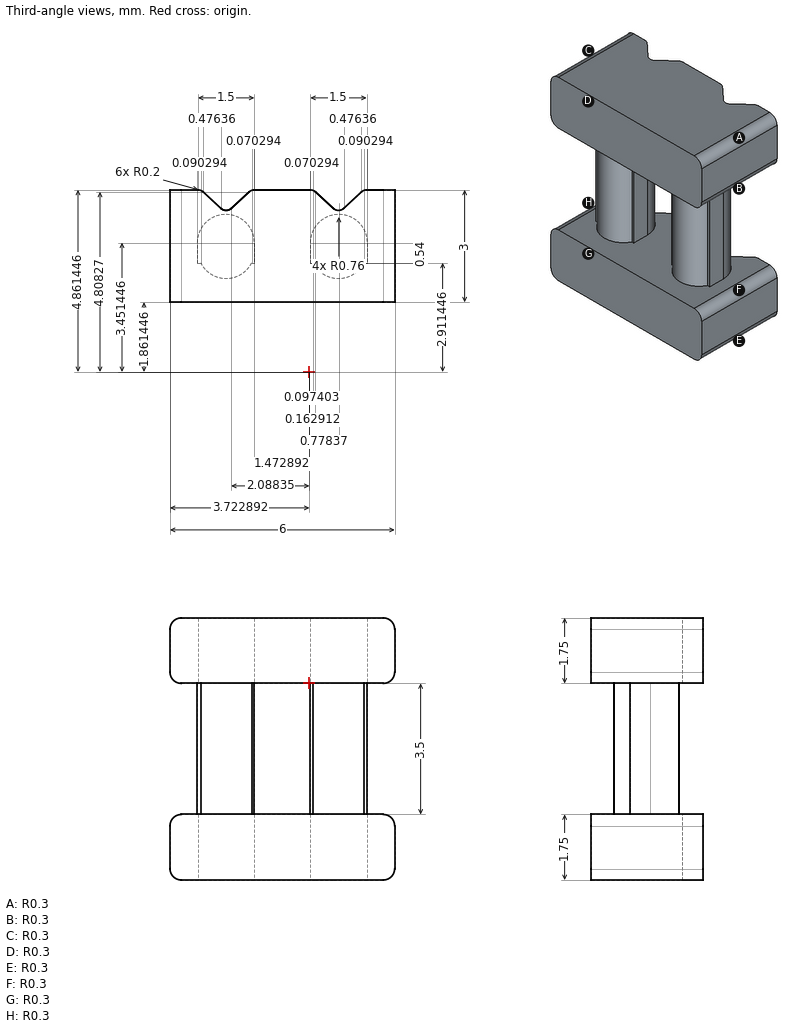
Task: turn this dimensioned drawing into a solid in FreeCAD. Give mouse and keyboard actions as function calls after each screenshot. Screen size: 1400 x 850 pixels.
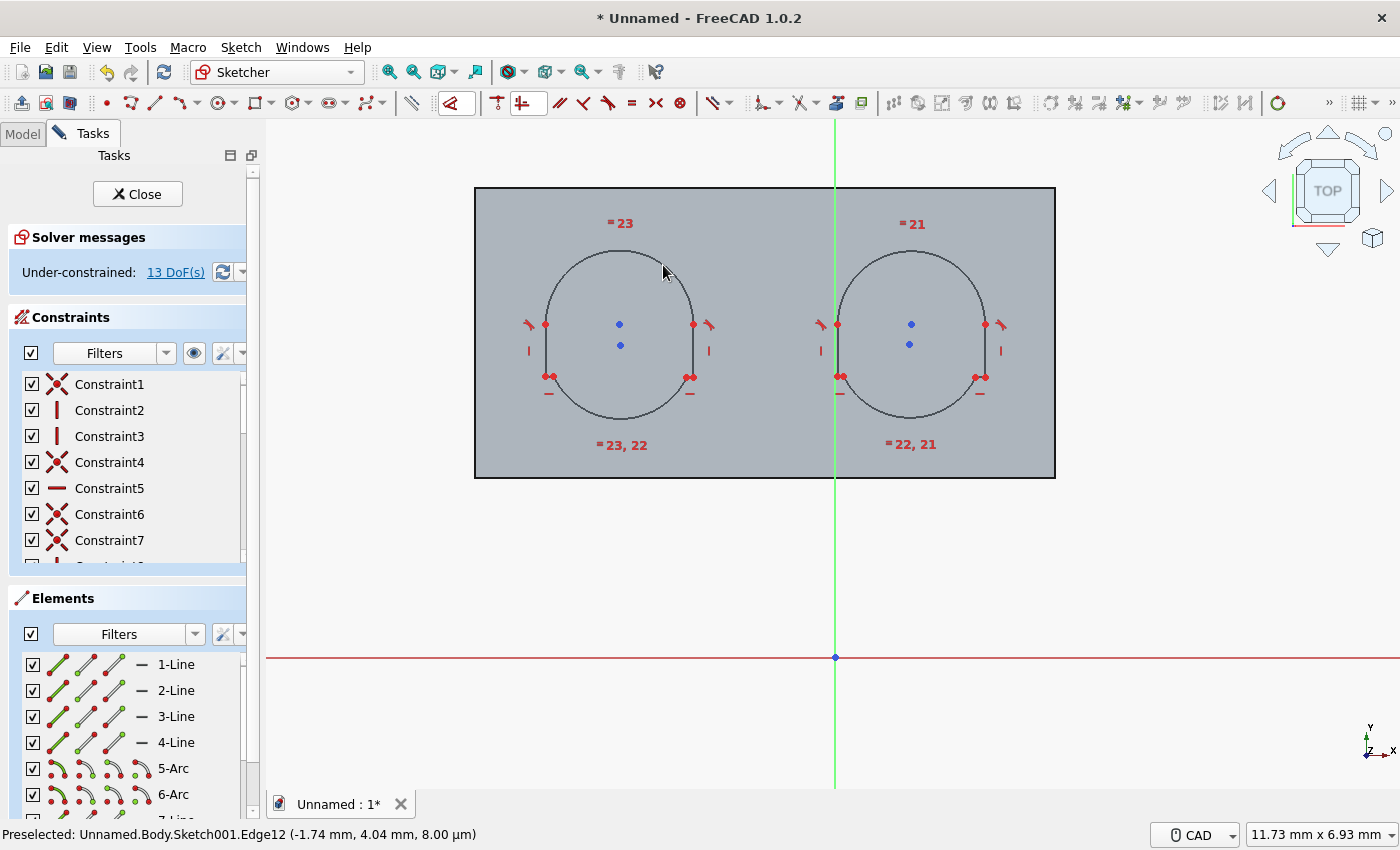
click(955, 265)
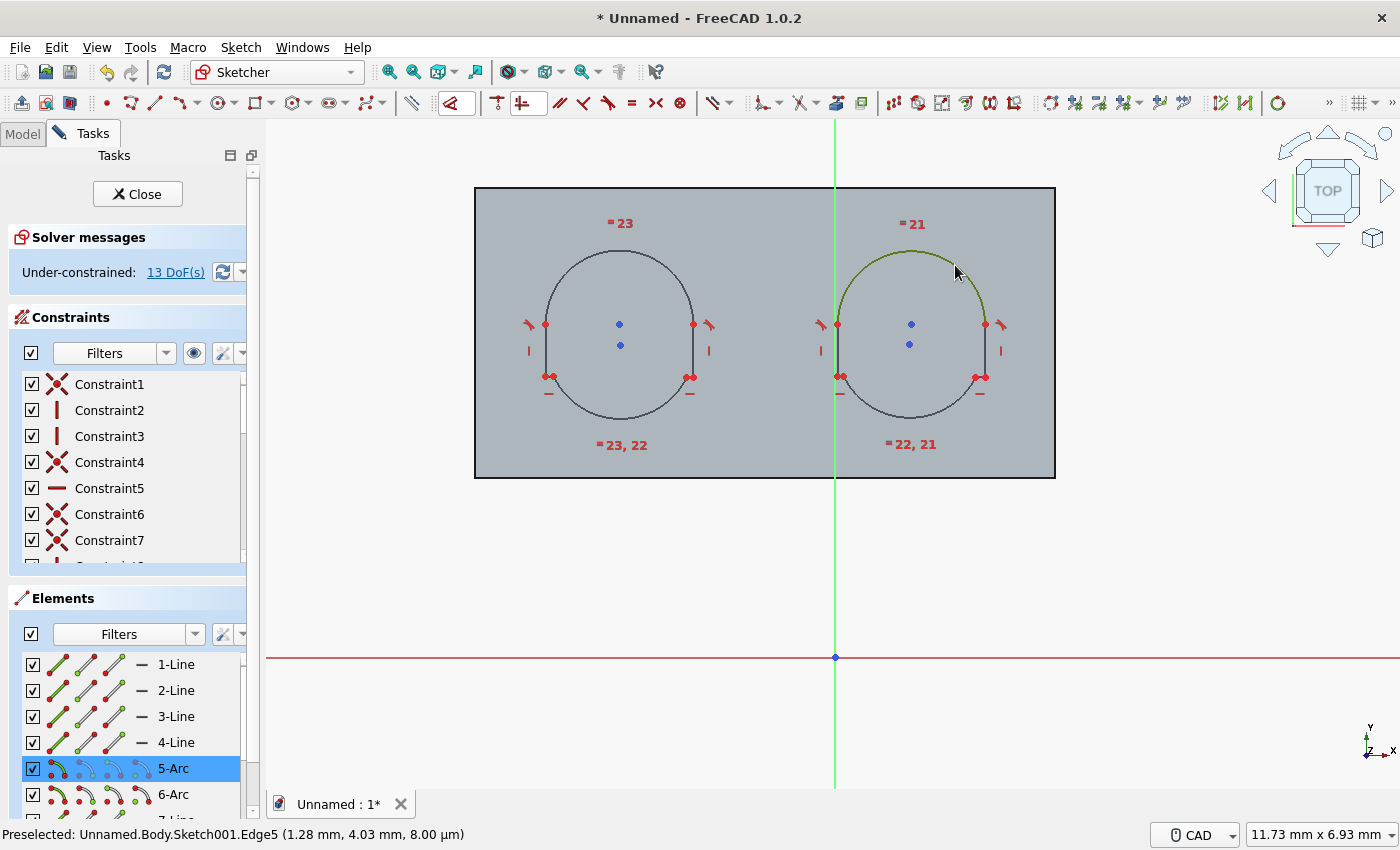
key(k)
key(r)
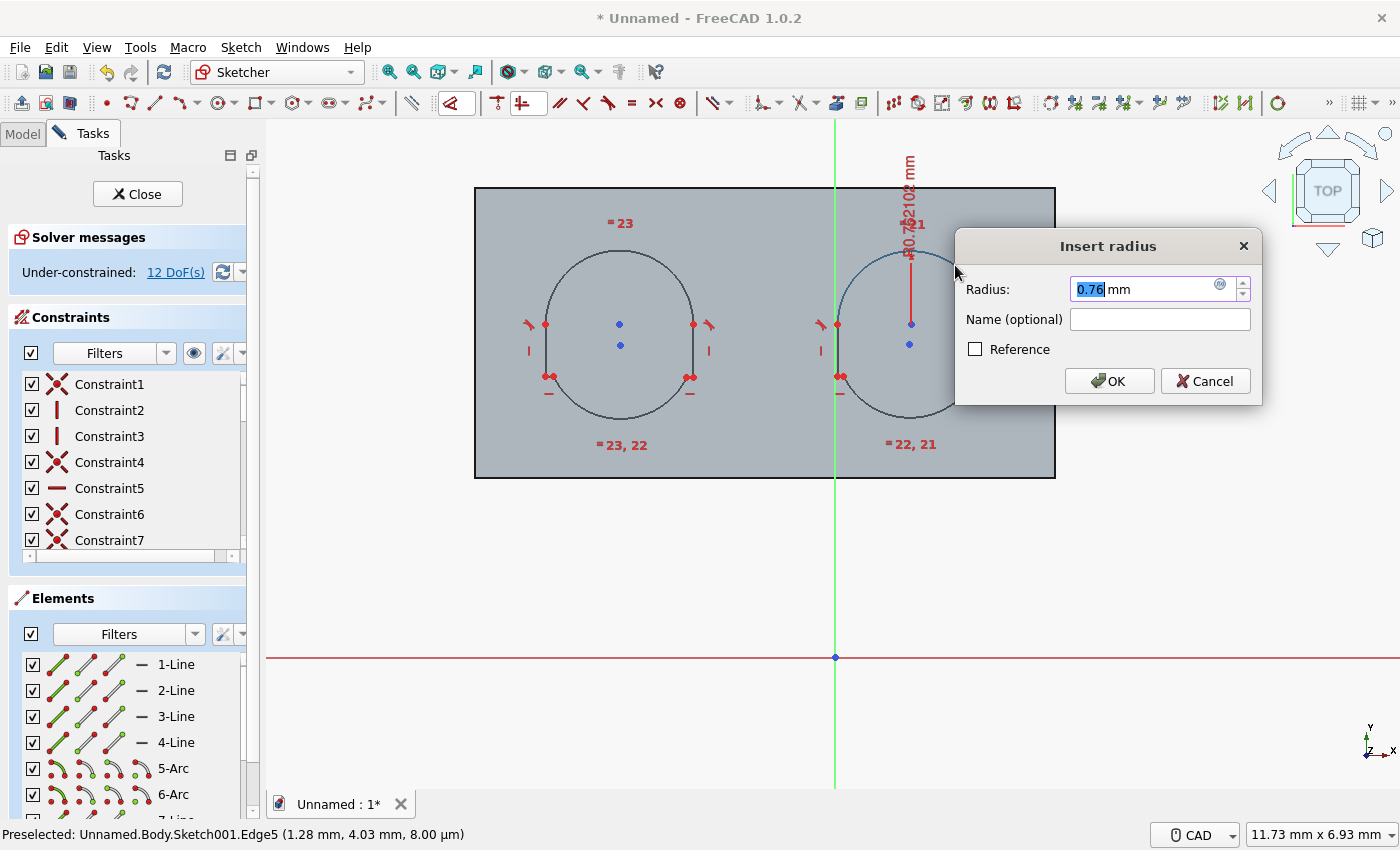
text(0.76)
key(Return)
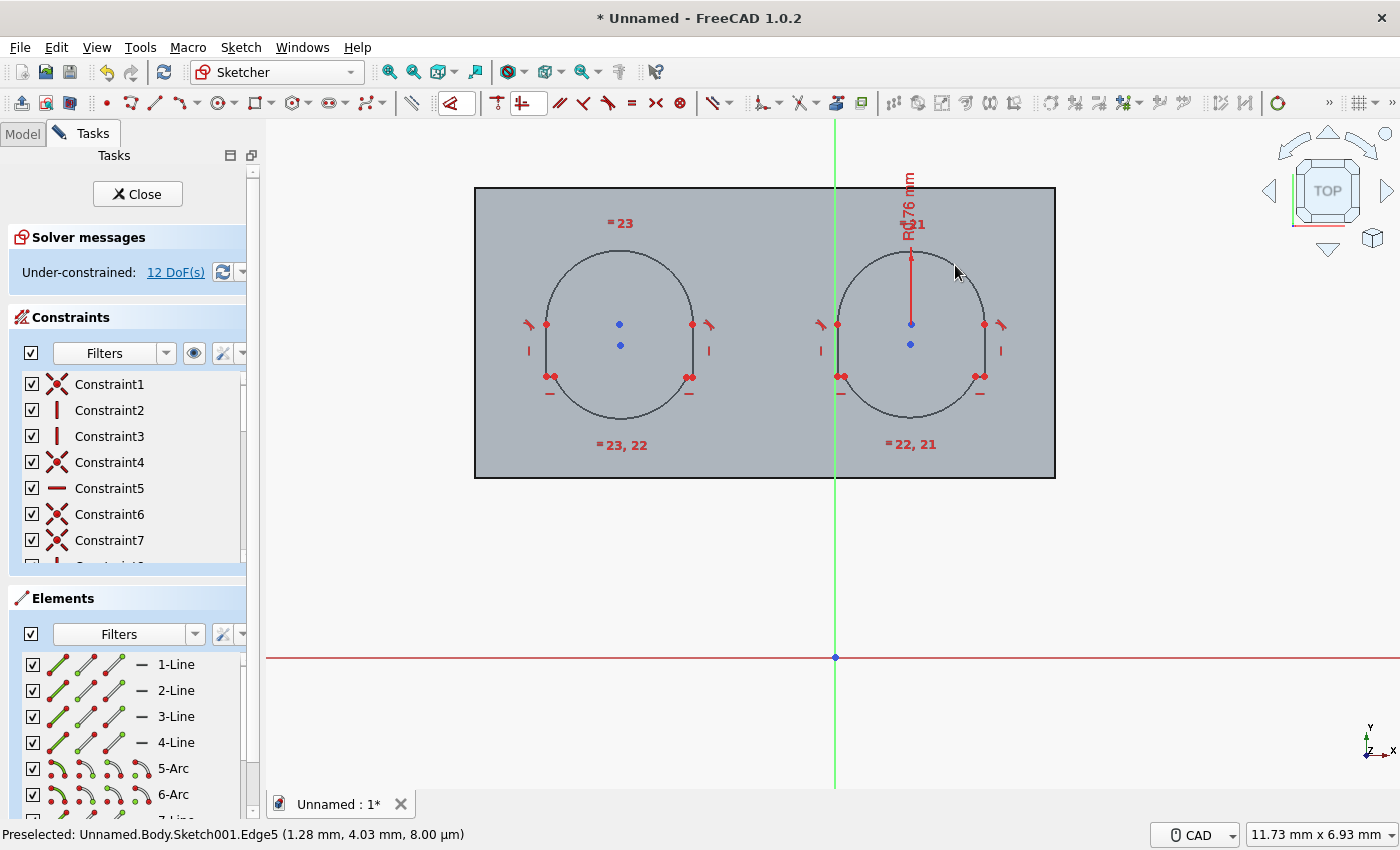
click(838, 361)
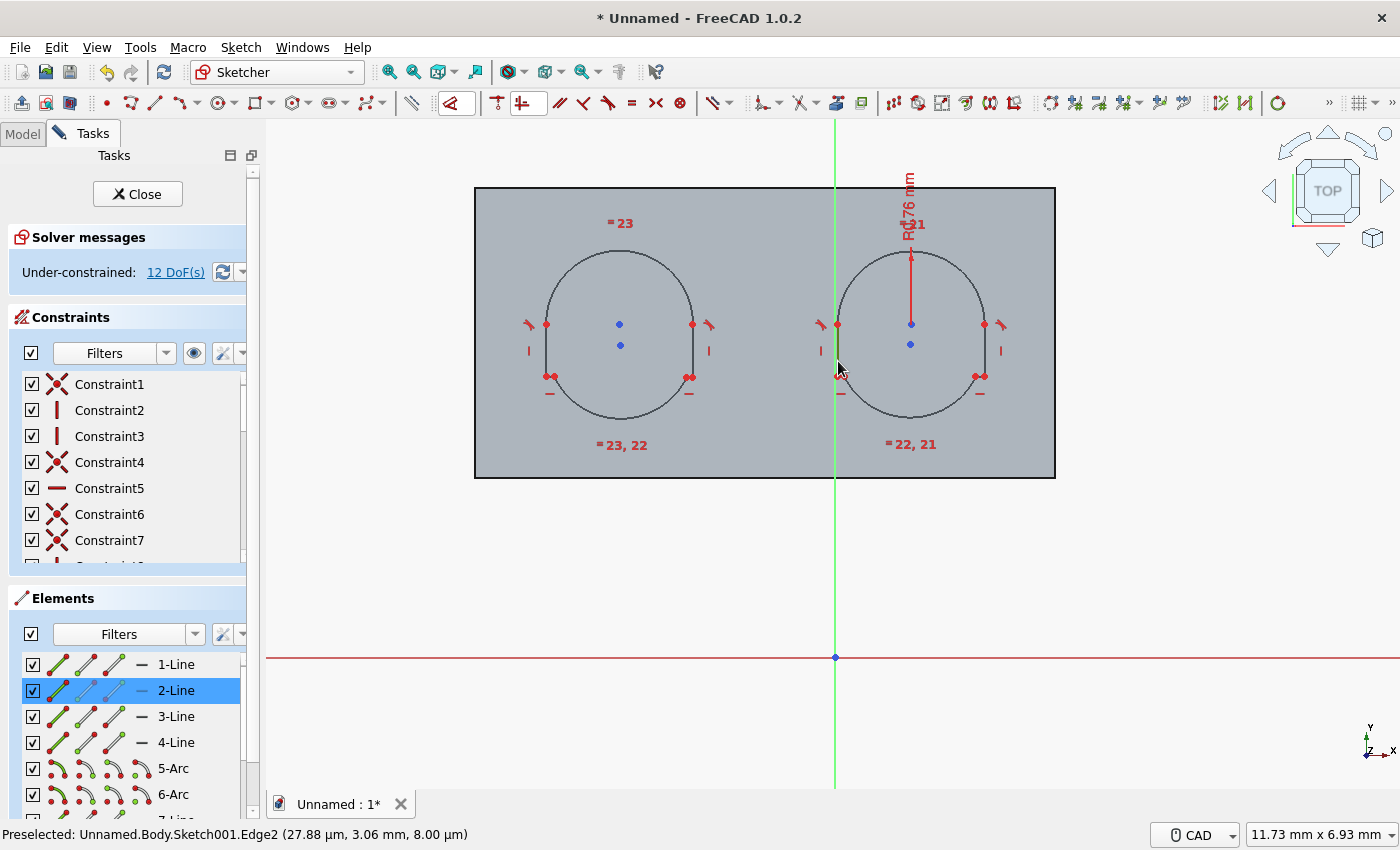
click(470, 104)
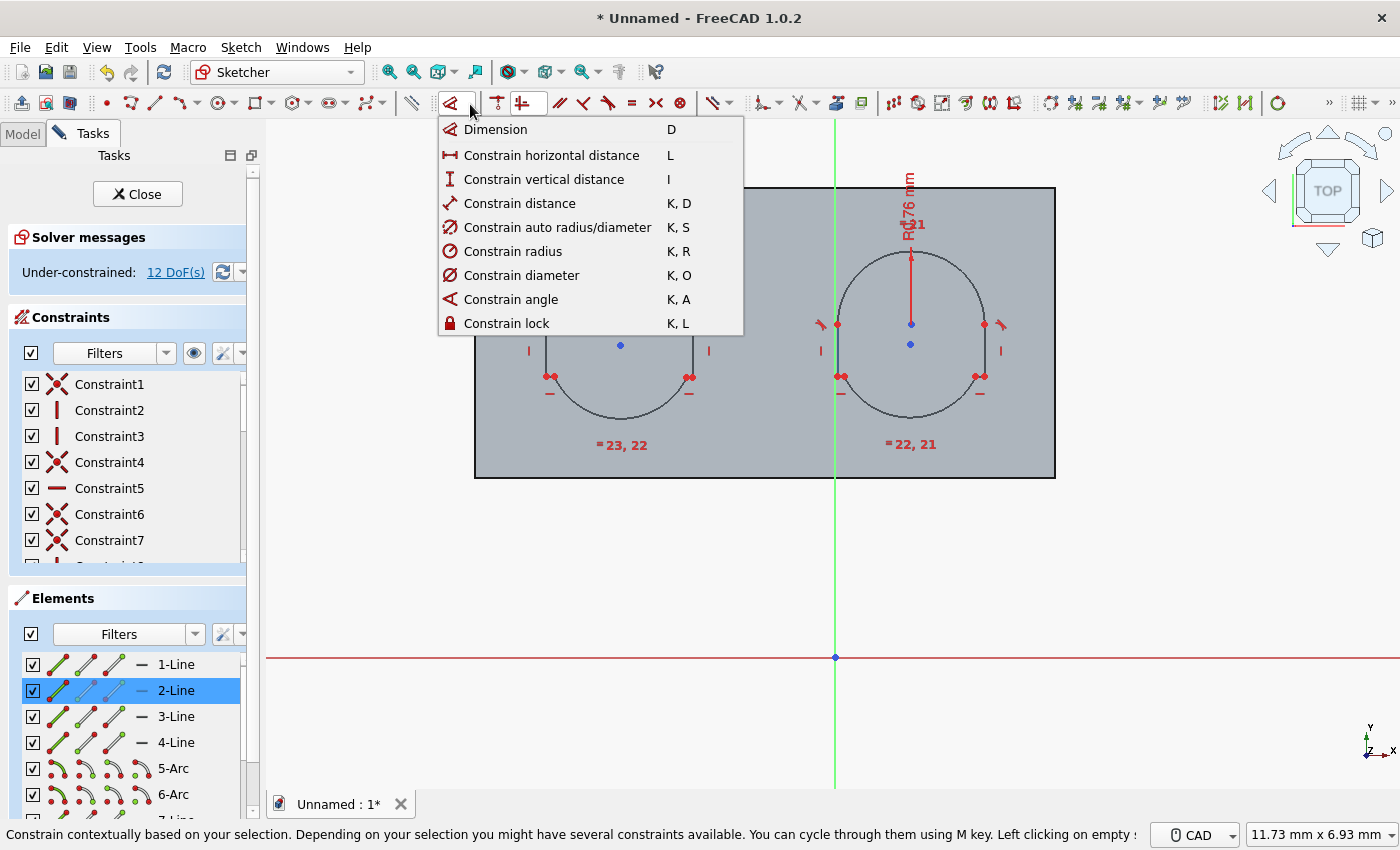
click(591, 179)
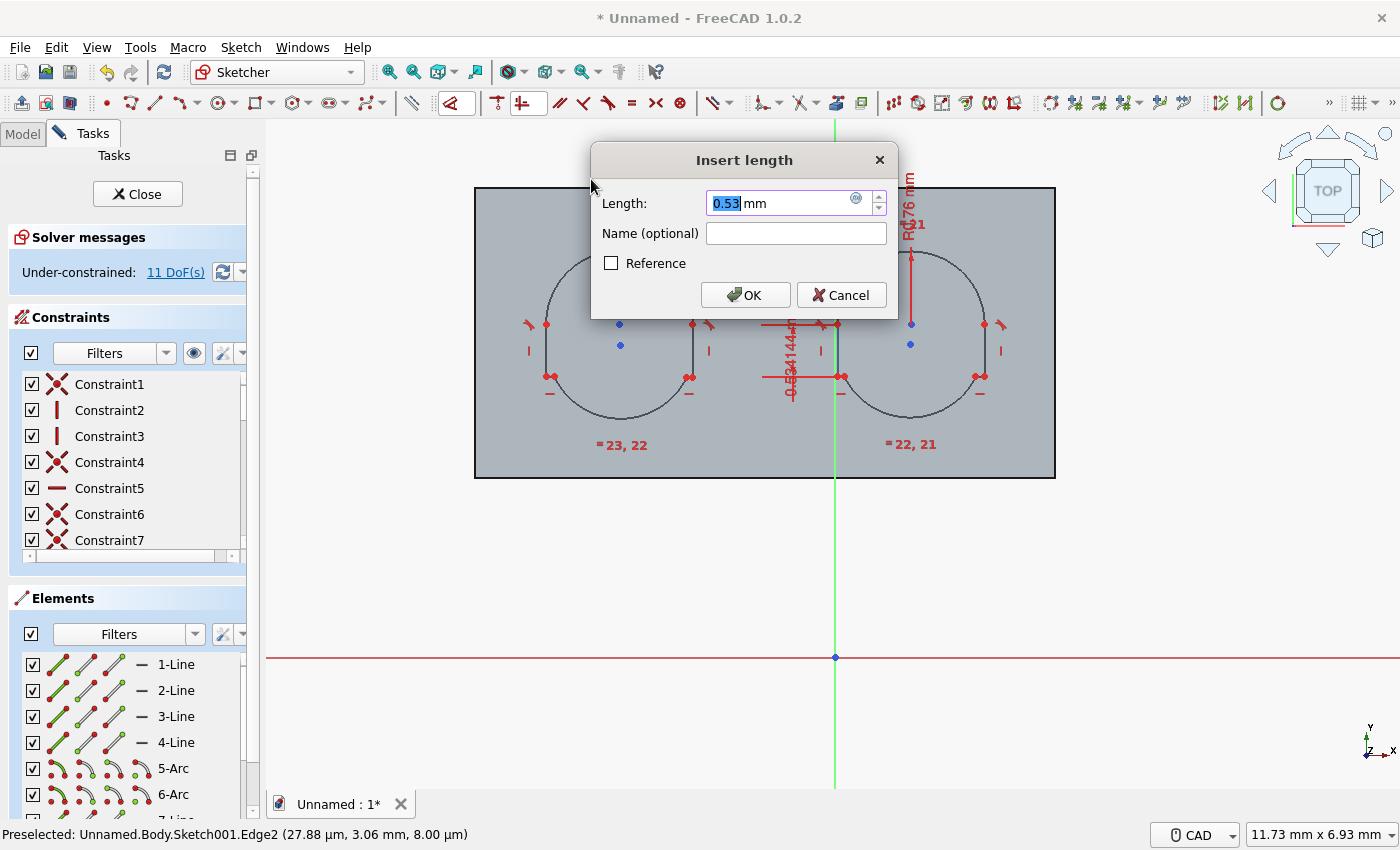
text(0.54)
key(Return)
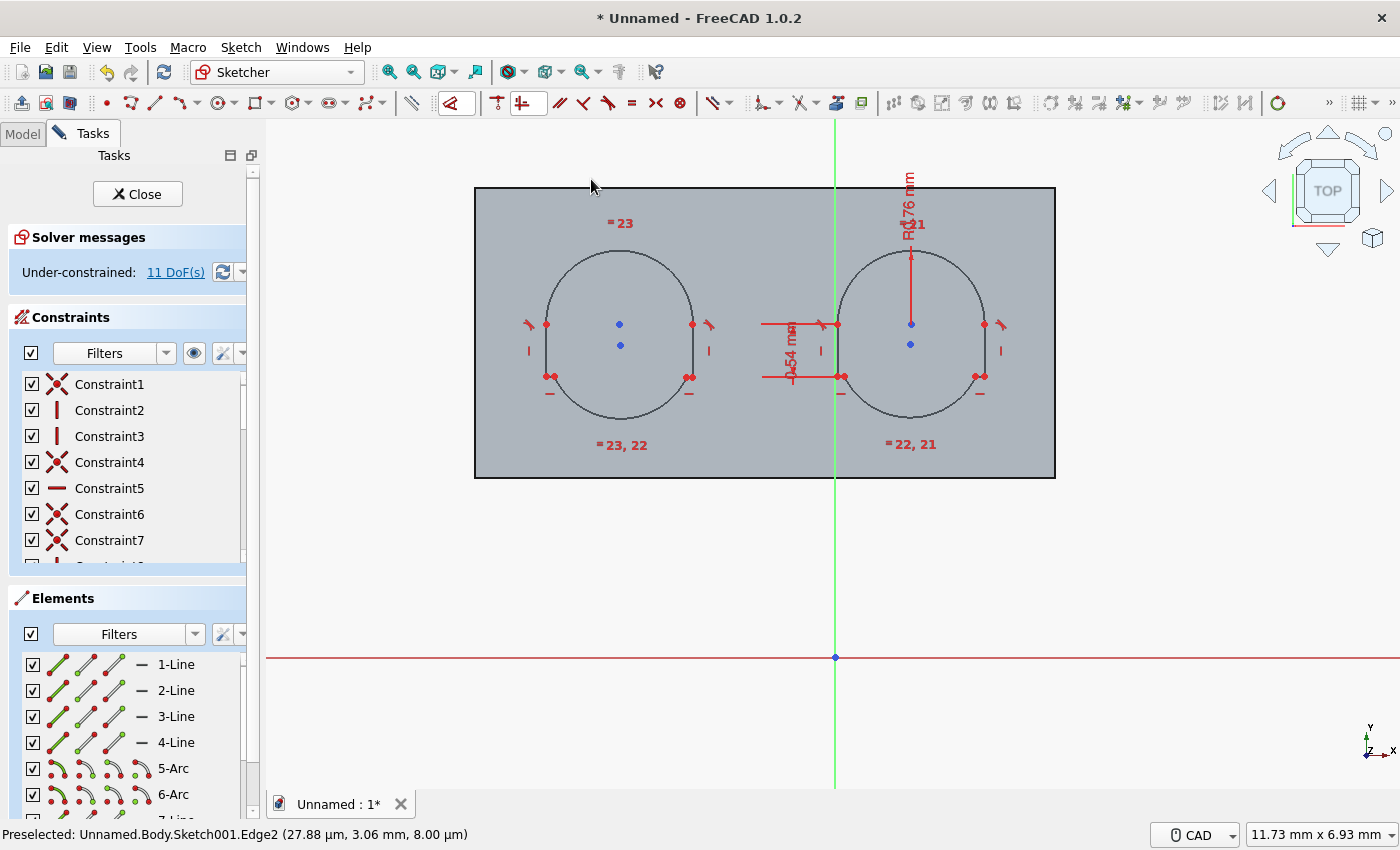
click(985, 340)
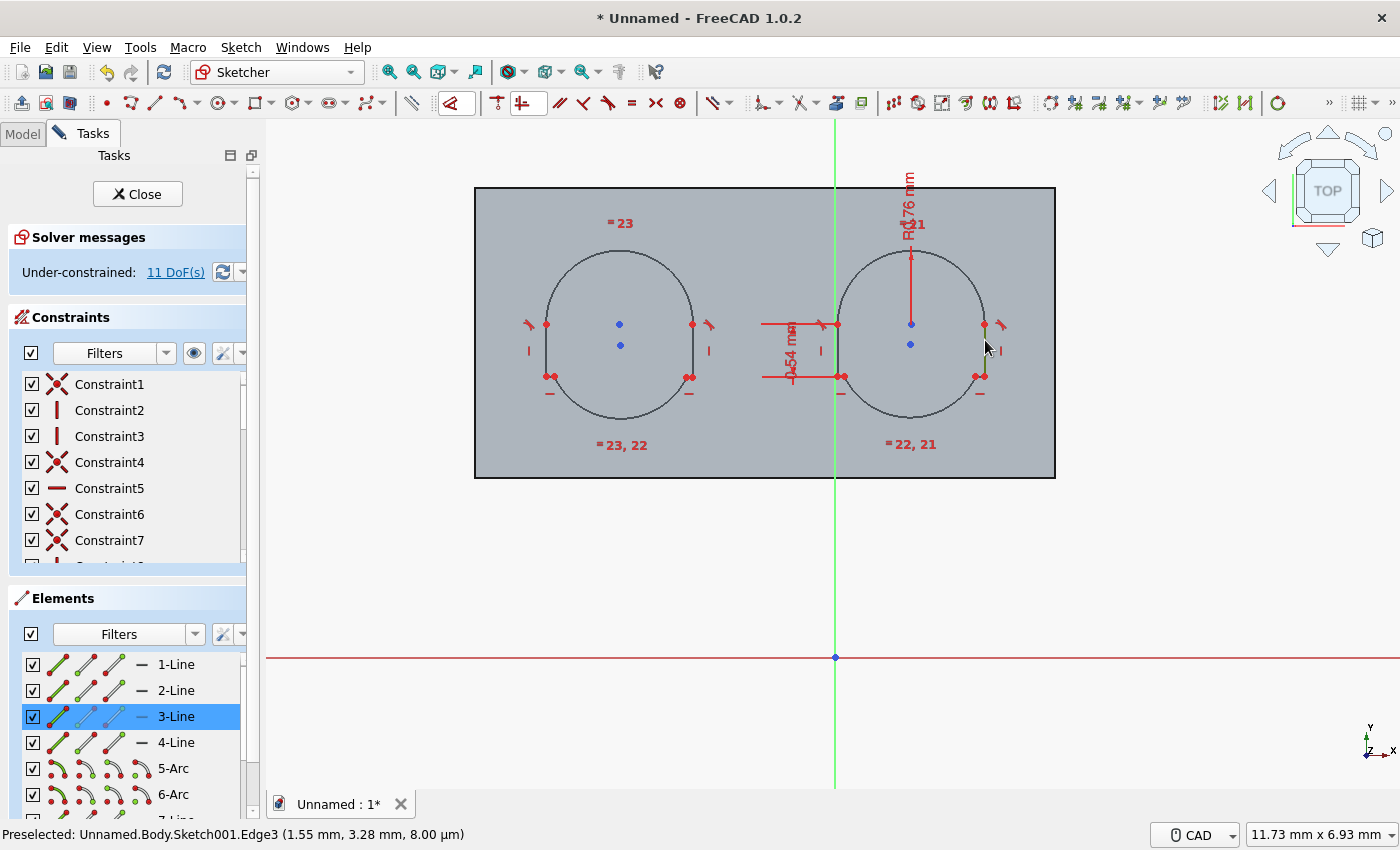
key(i)